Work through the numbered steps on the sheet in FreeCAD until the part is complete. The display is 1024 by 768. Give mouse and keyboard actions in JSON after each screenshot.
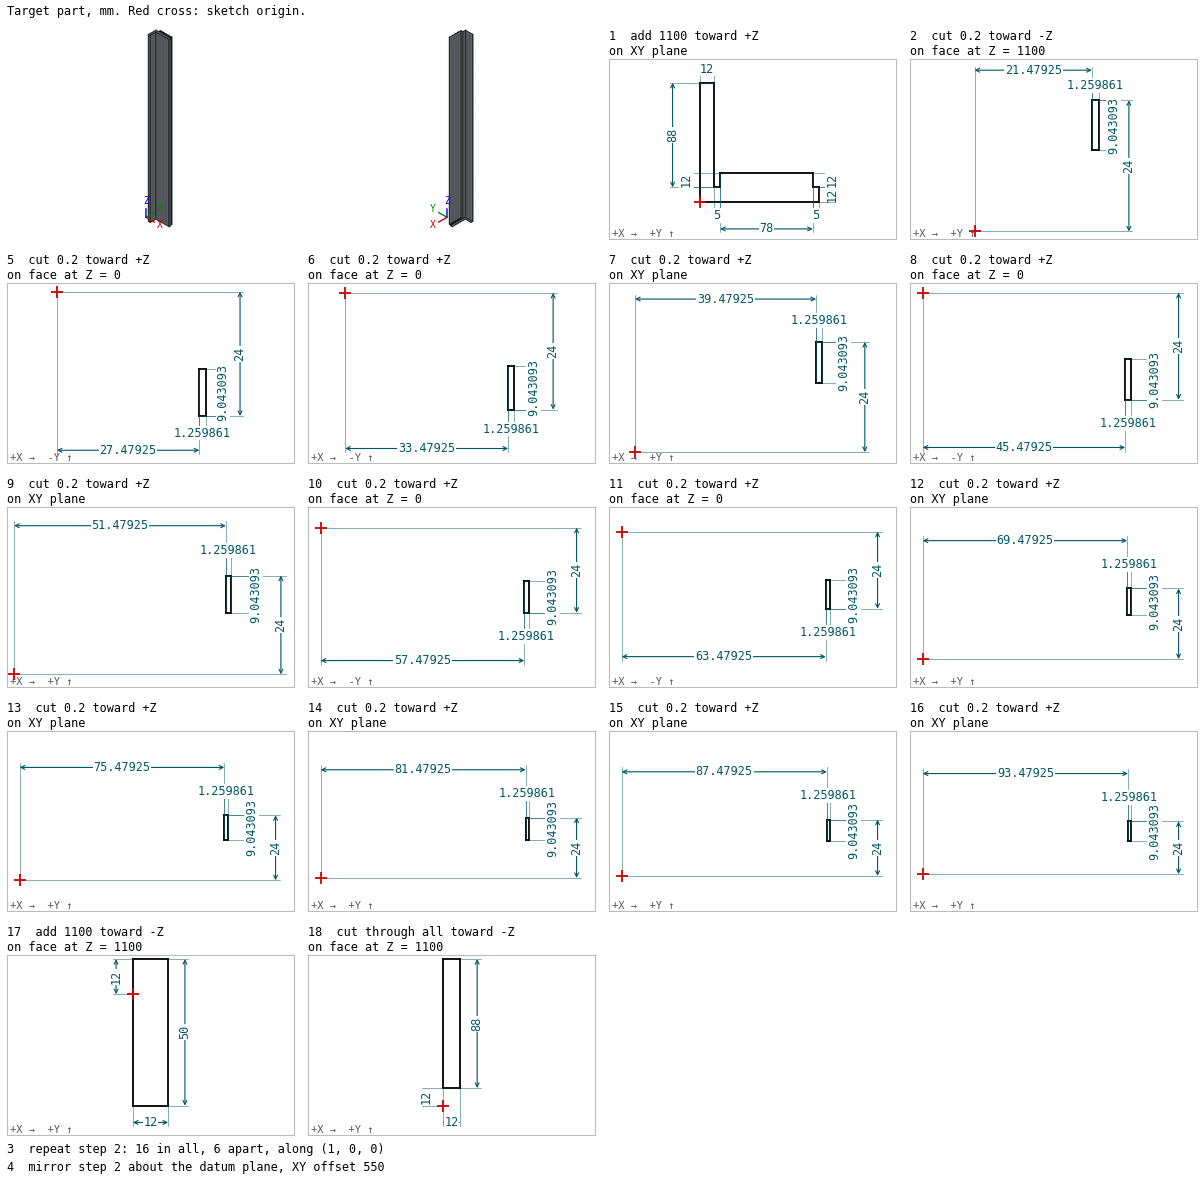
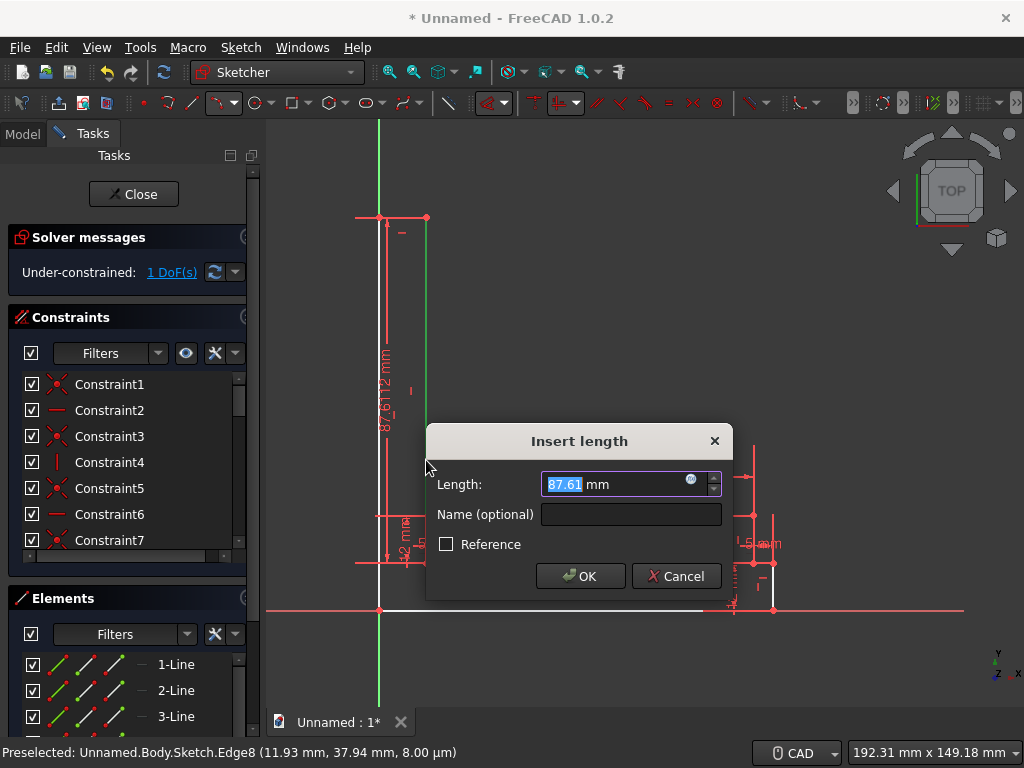
{"action": "type", "text": "88"}
{"action": "key", "text": "Return"}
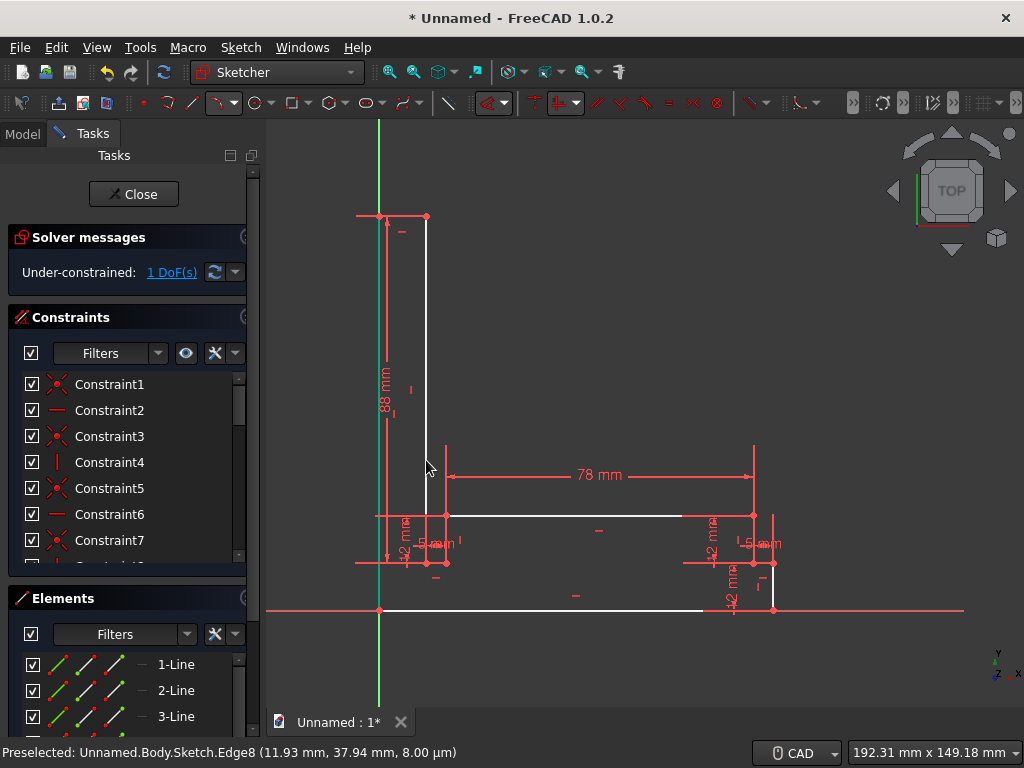
{"action": "left_click", "coordinate": [412, 216]}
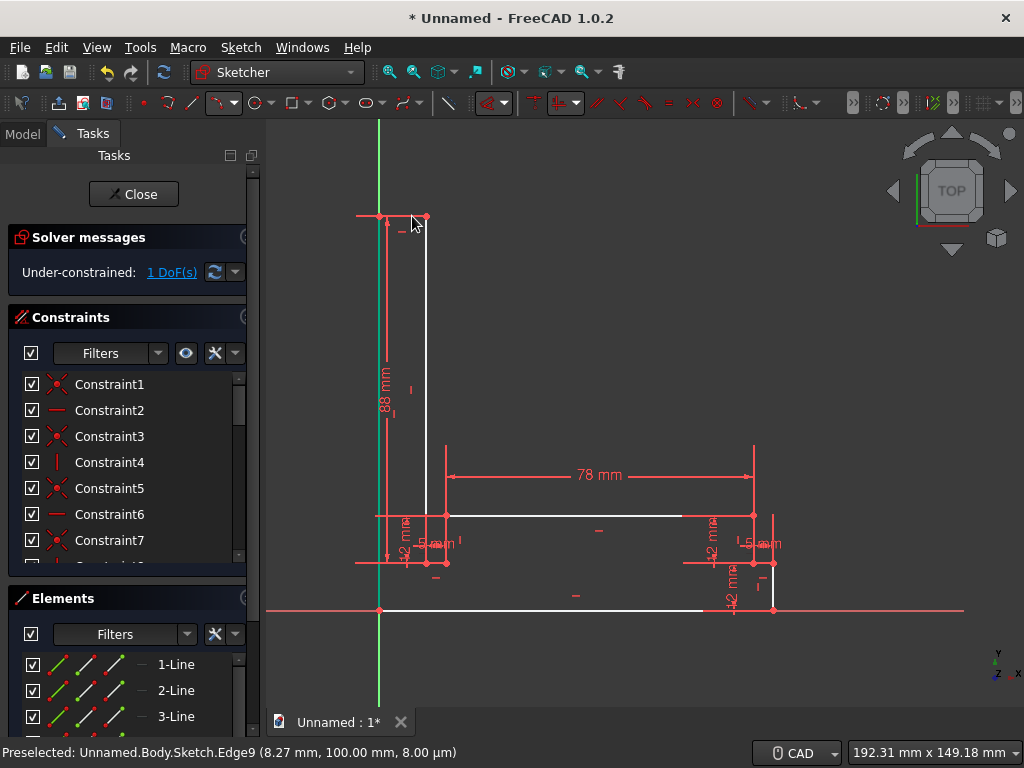
{"action": "key", "text": "l"}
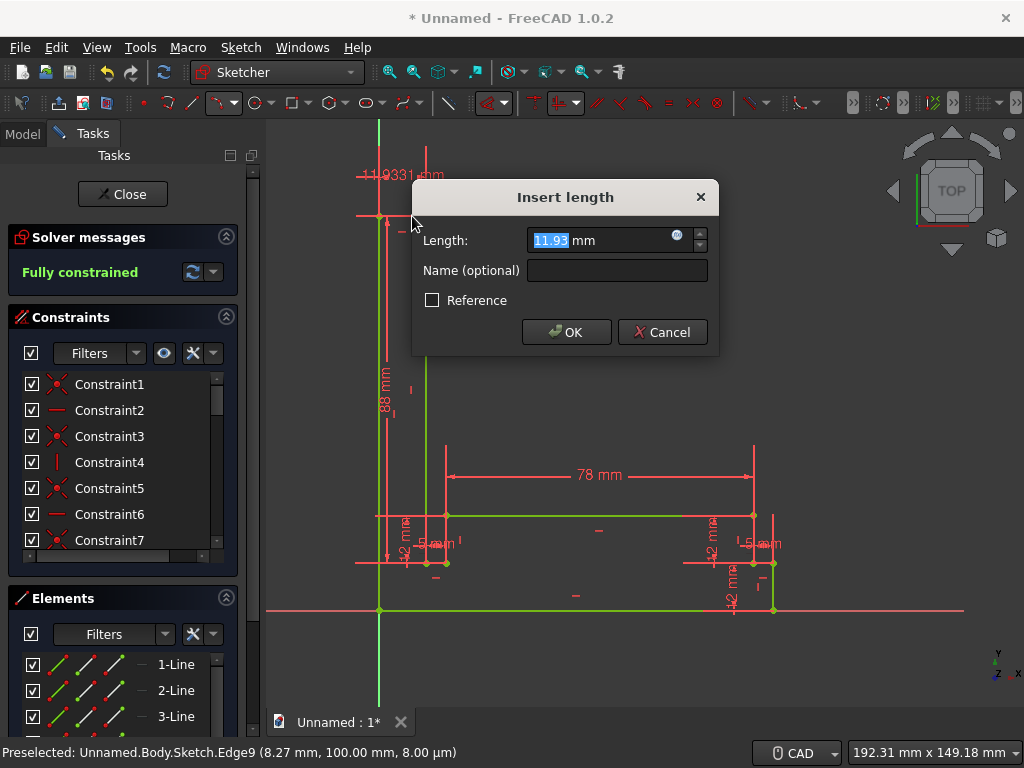
{"action": "type", "text": "12"}
{"action": "key", "text": "Return"}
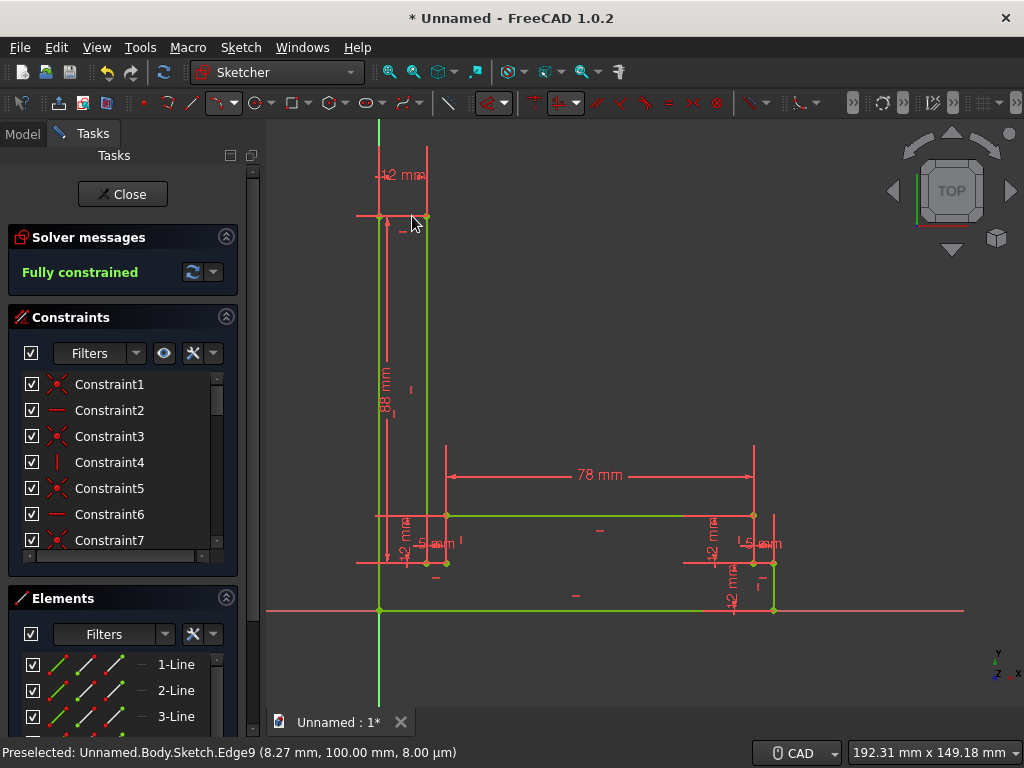
{"action": "left_click", "coordinate": [123, 194]}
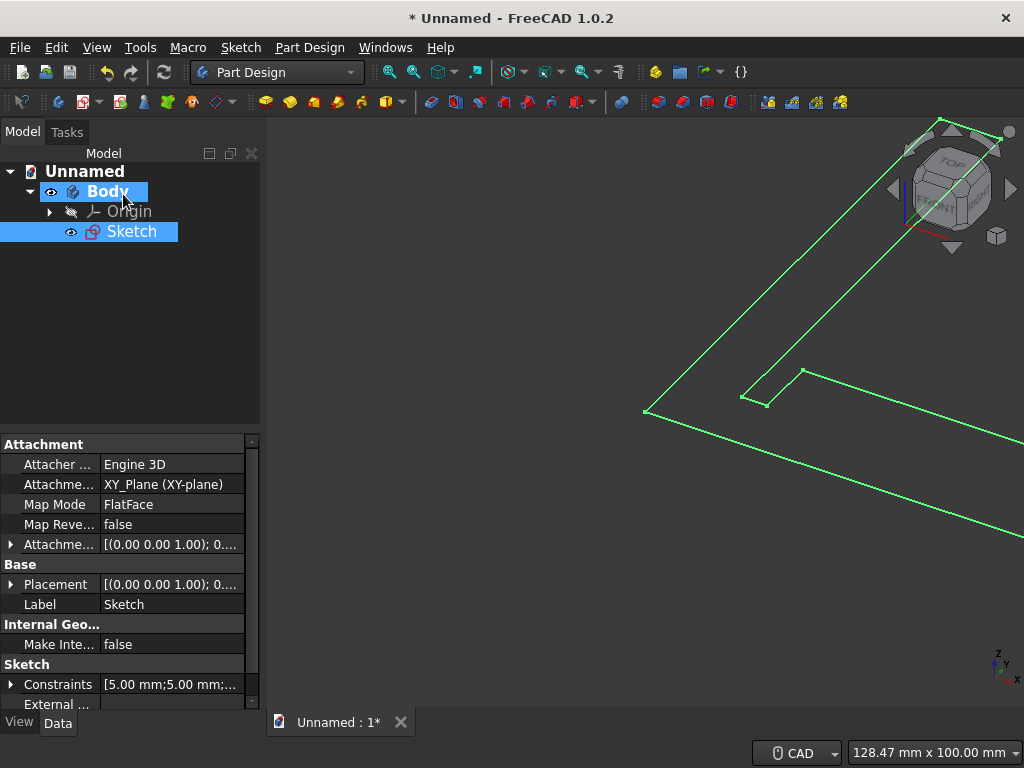
{"action": "left_click", "coordinate": [266, 102]}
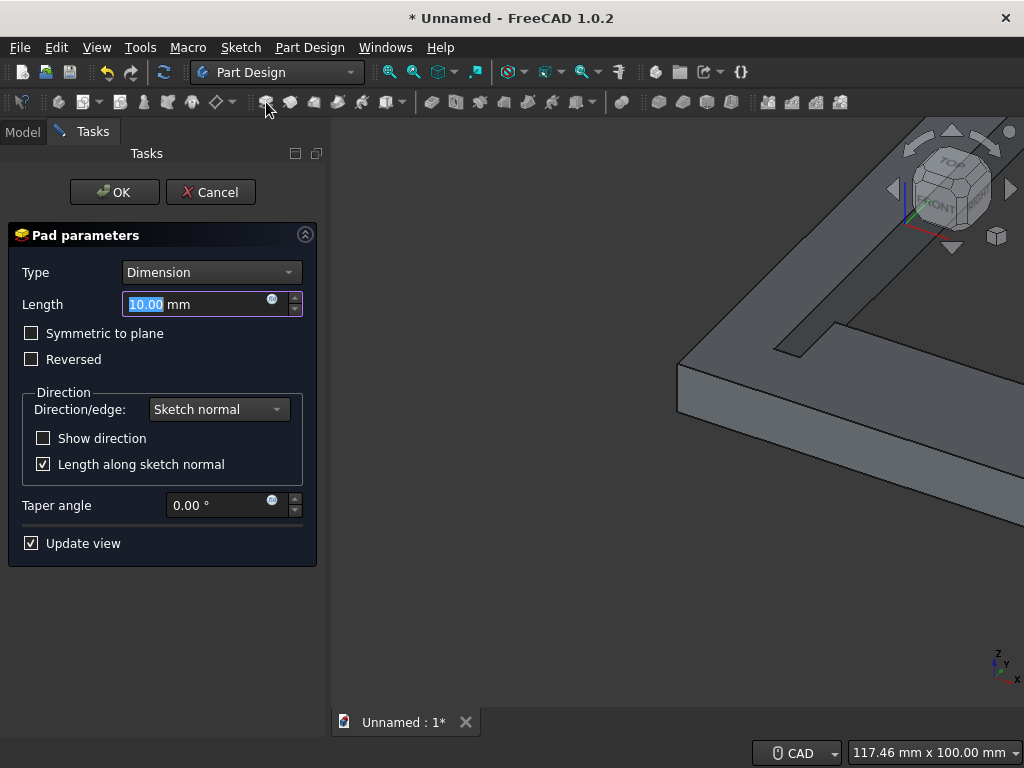
{"action": "type", "text": "1100"}
{"action": "key", "text": "Tab"}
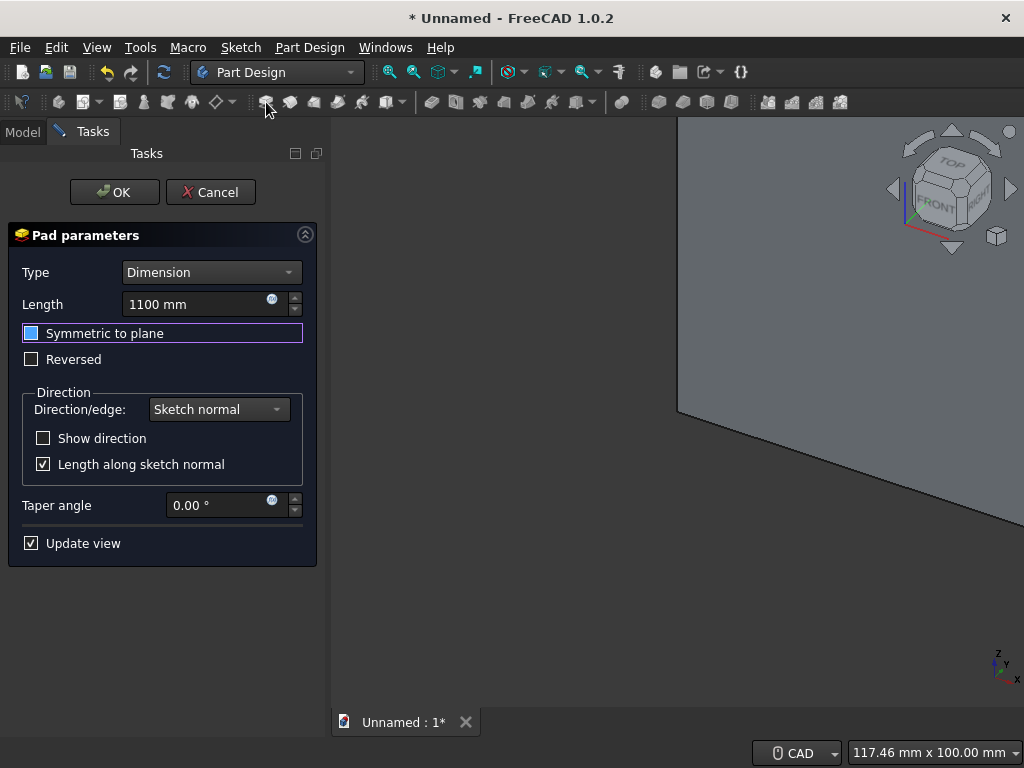
{"action": "left_click", "coordinate": [115, 192]}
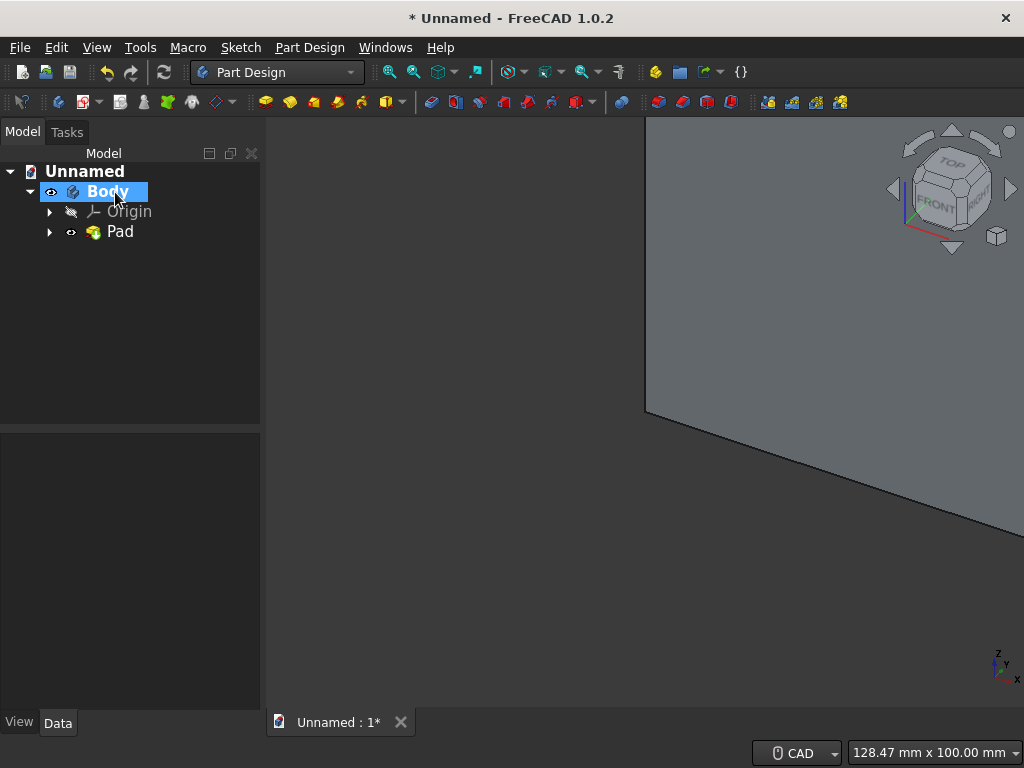
{"action": "left_click", "coordinate": [390, 72]}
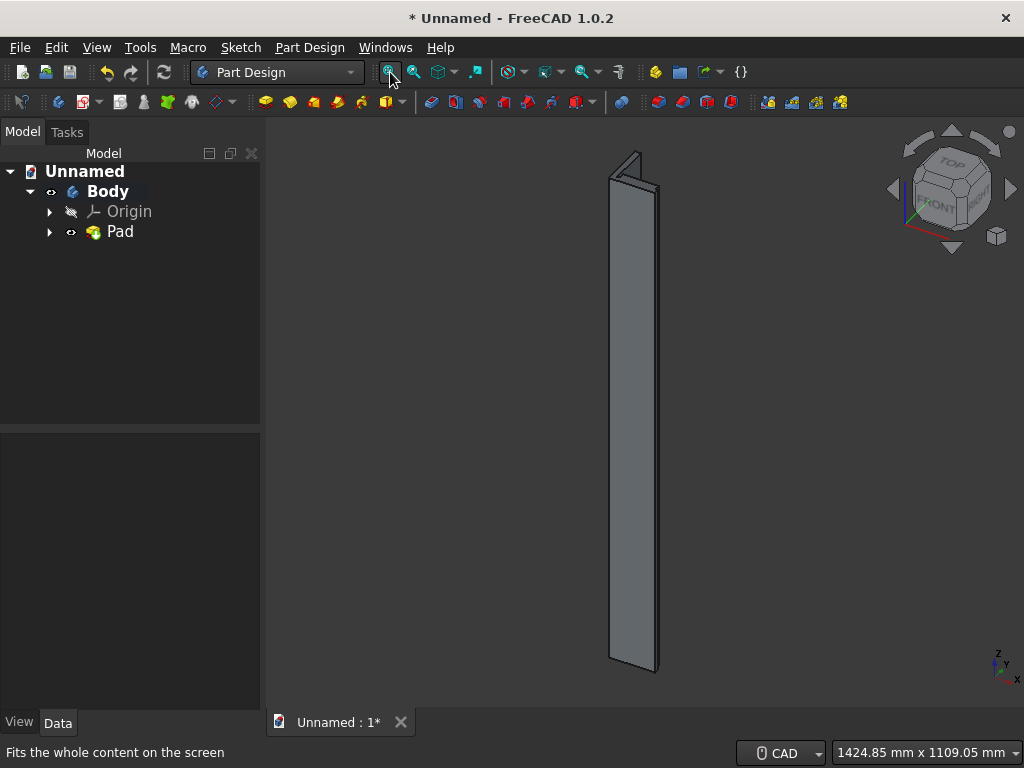
{"action": "scroll", "coordinate": [647, 187], "scroll_direction": "up", "scroll_amount": 6}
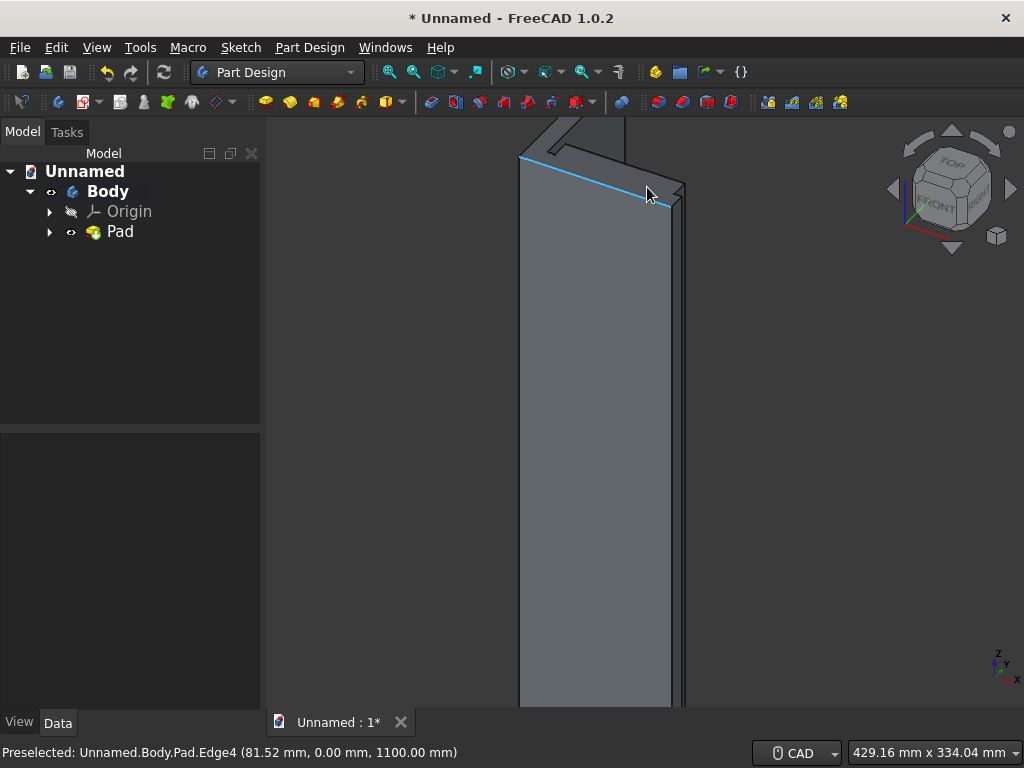
{"action": "key", "text": "v f"}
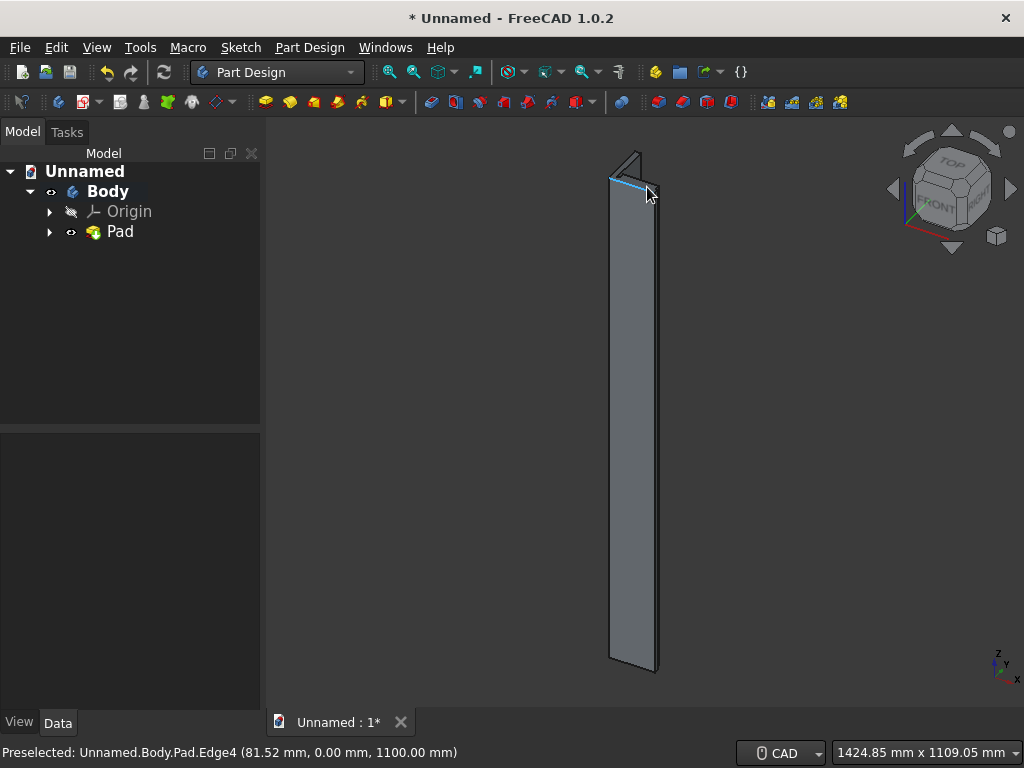
{"action": "key", "text": "0"}